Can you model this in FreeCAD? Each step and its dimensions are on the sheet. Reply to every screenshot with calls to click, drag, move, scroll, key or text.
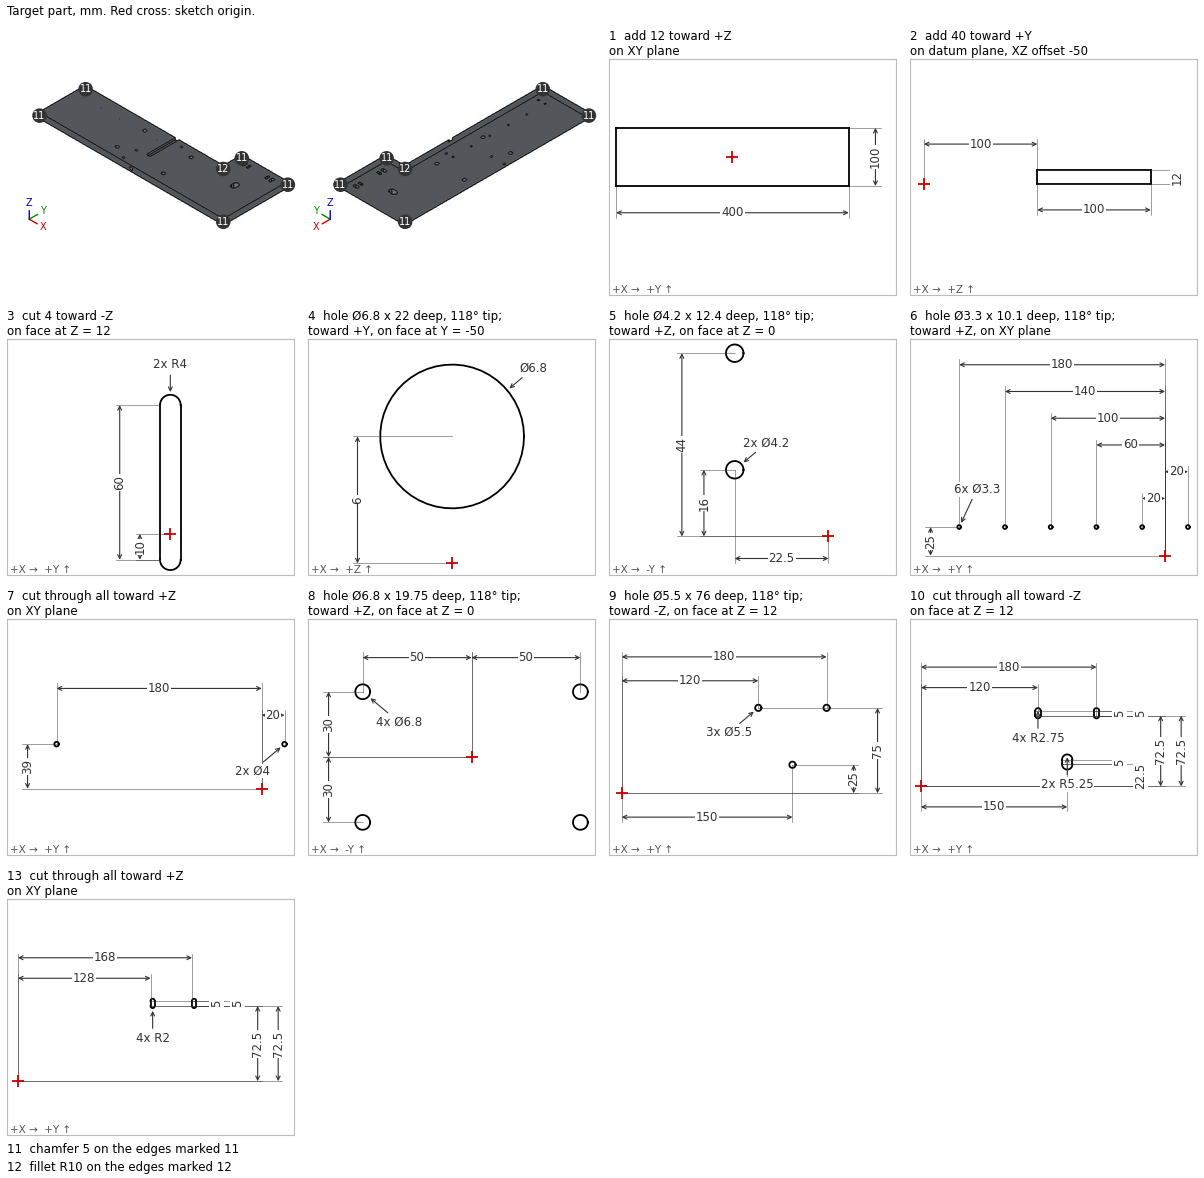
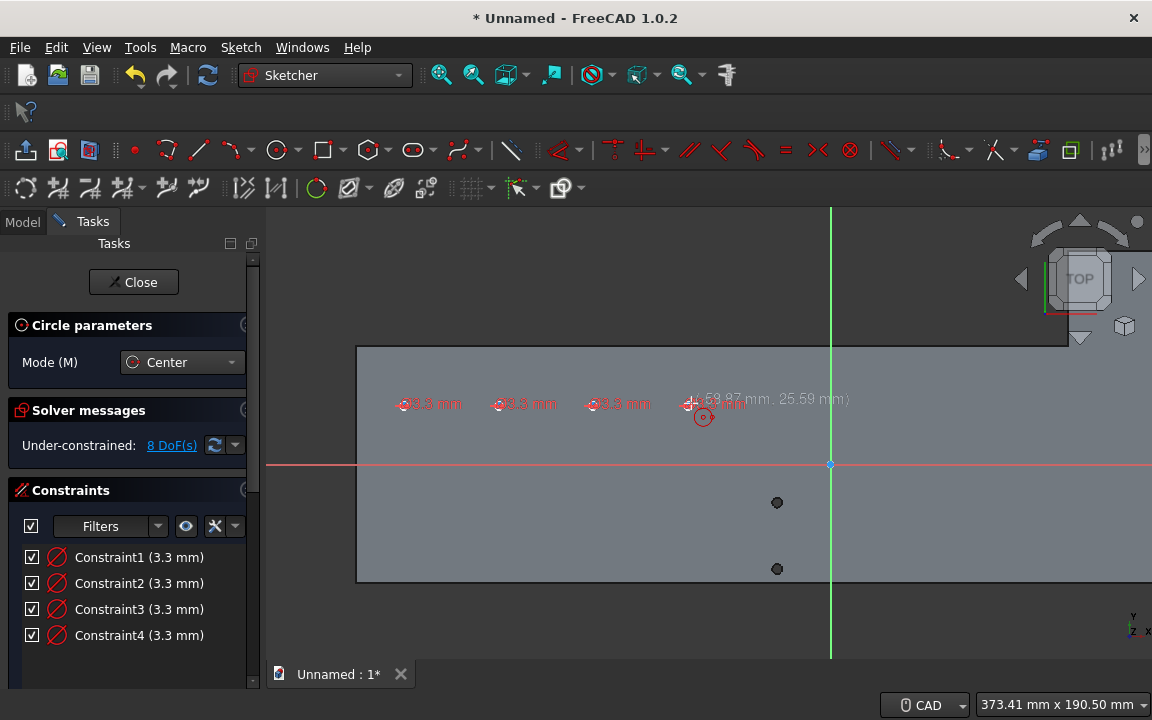
scroll(783, 405, up, 9)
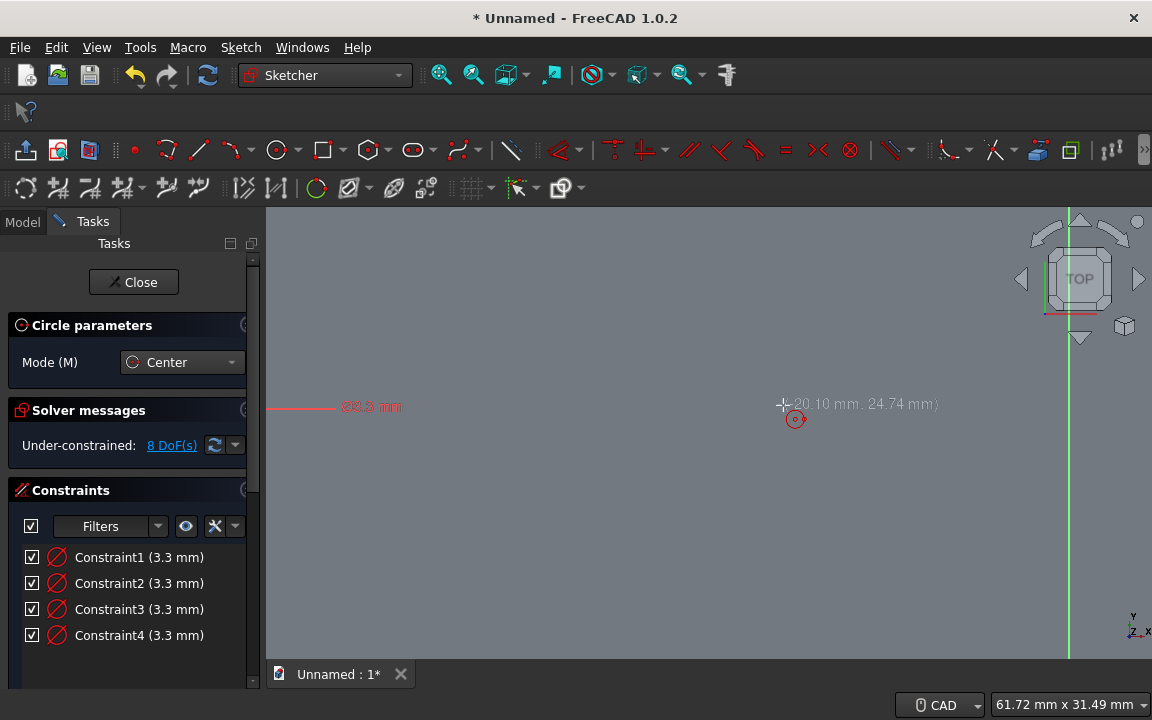
scroll(783, 405, down, 9)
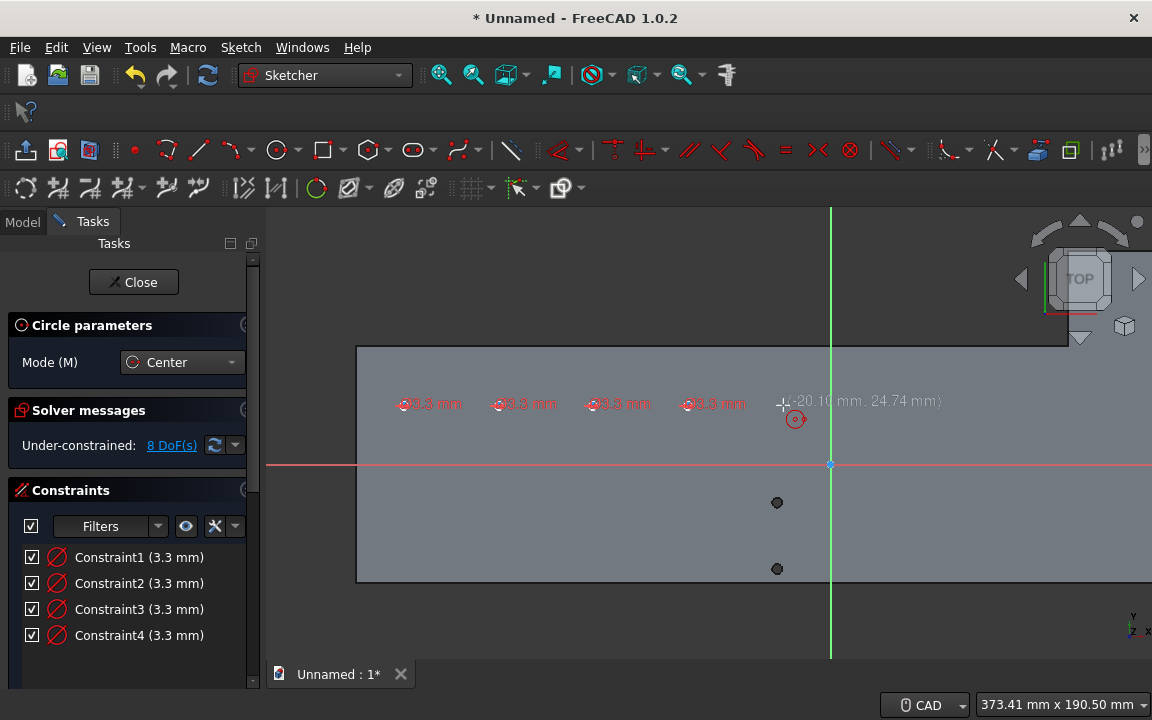
click(783, 405)
move(786, 403)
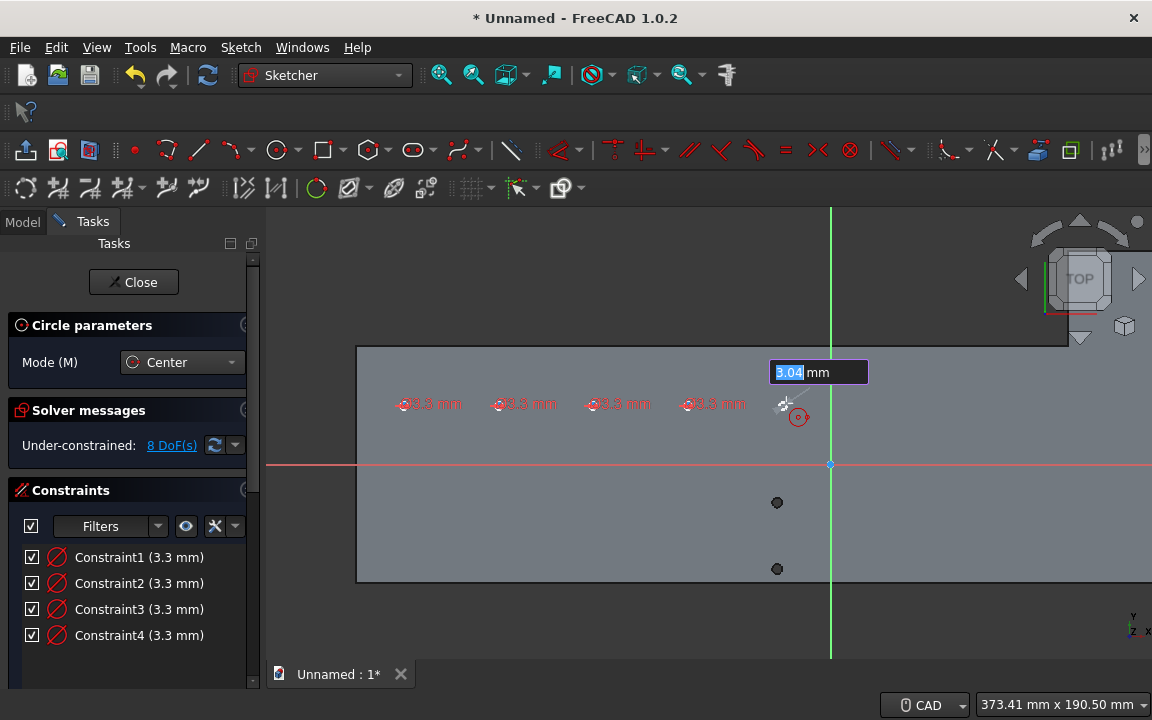
text(3.3)
key(Return)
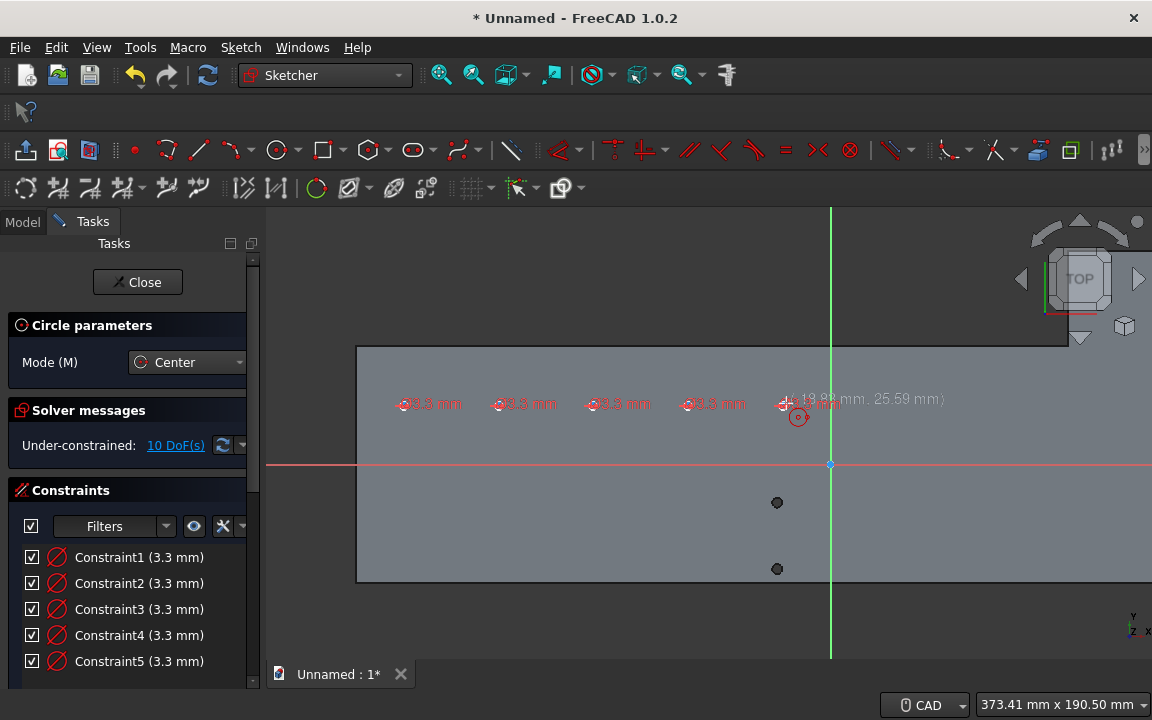
scroll(878, 405, up, 9)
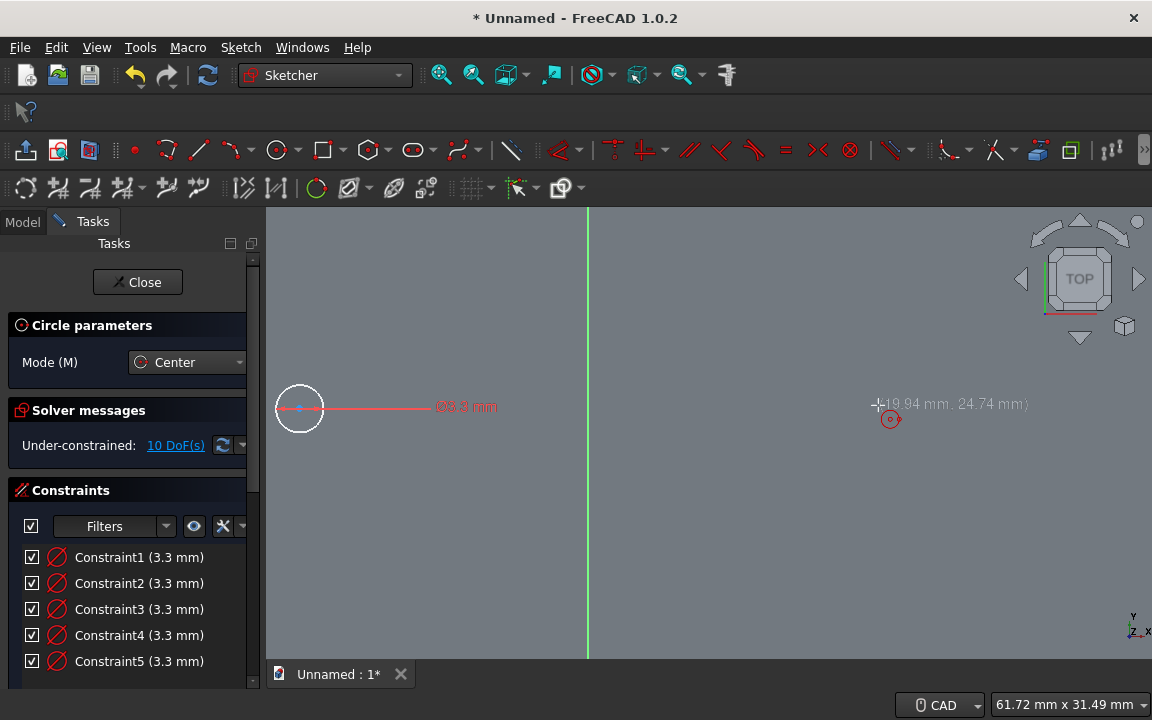
scroll(878, 405, down, 9)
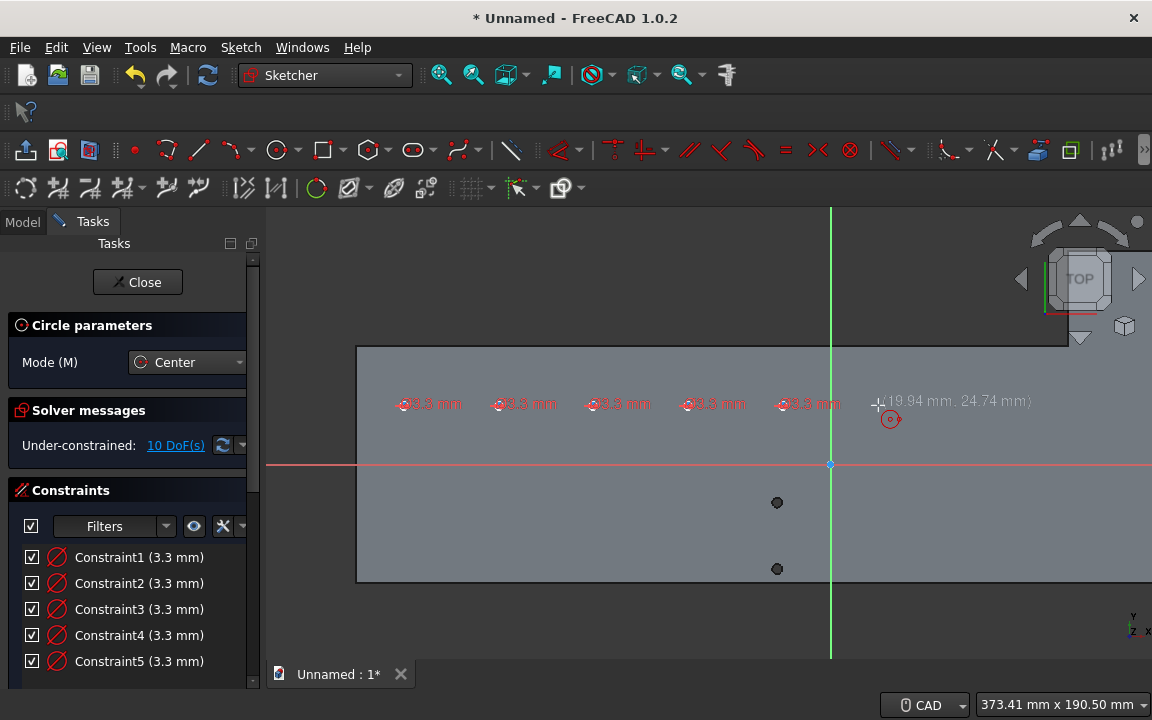
click(878, 405)
move(881, 403)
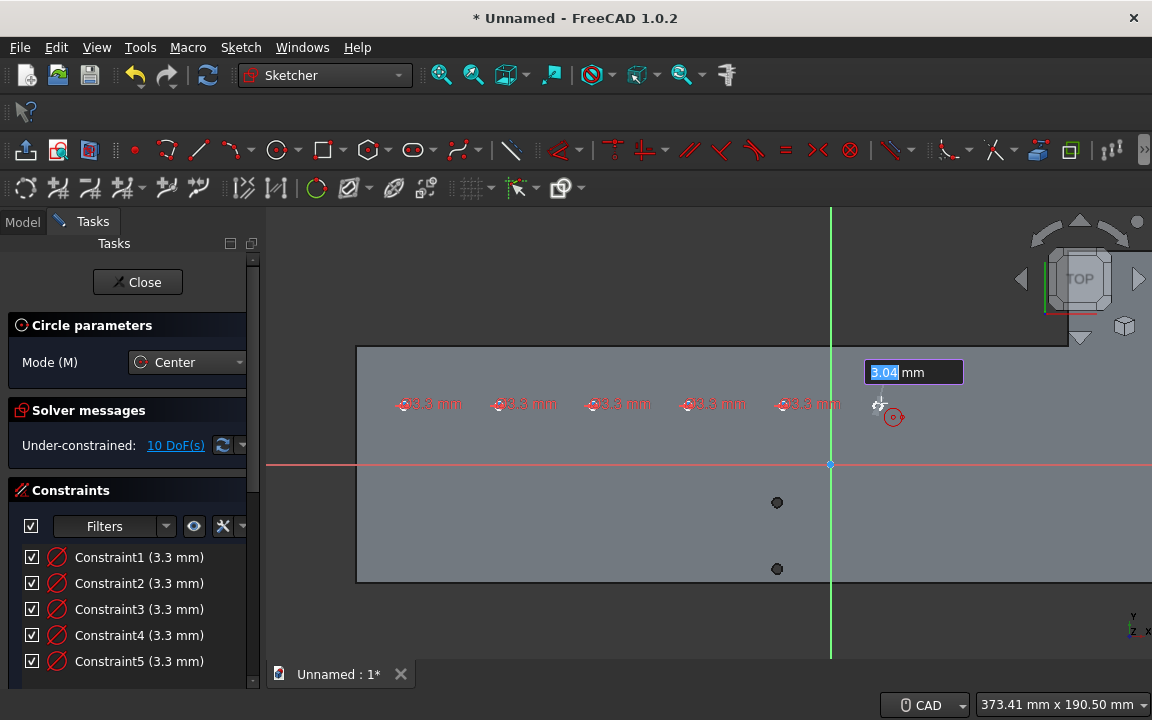
text(3.3)
key(Return)
key(Escape)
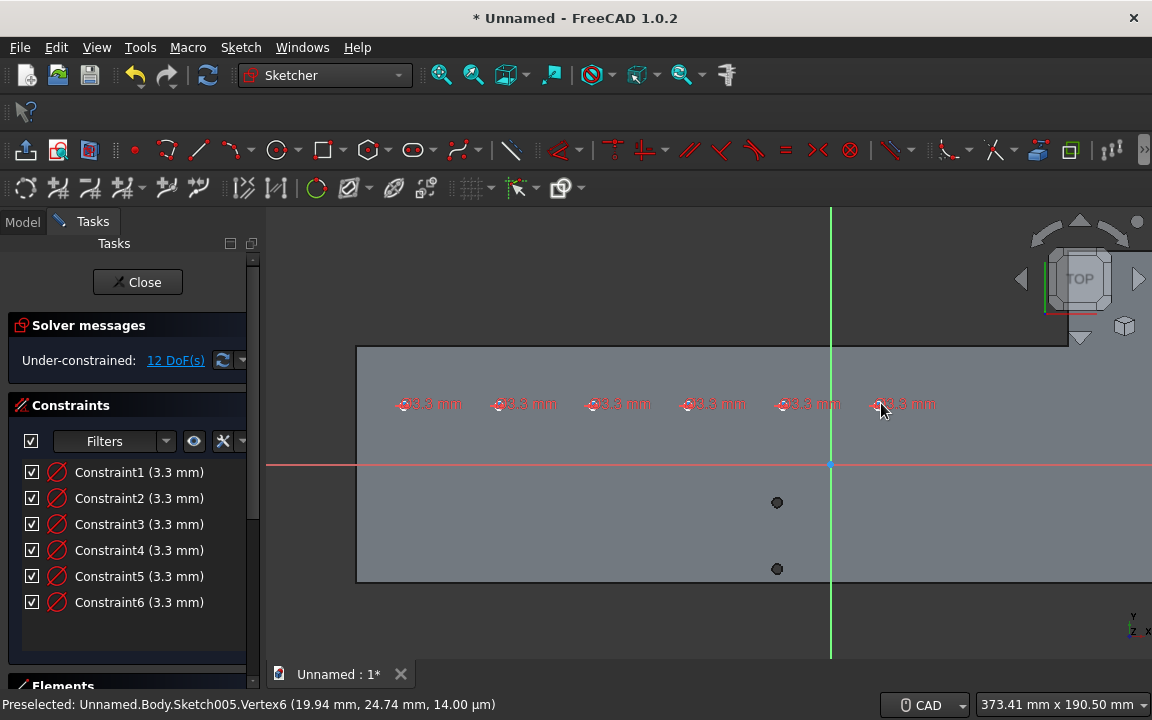
click(404, 406)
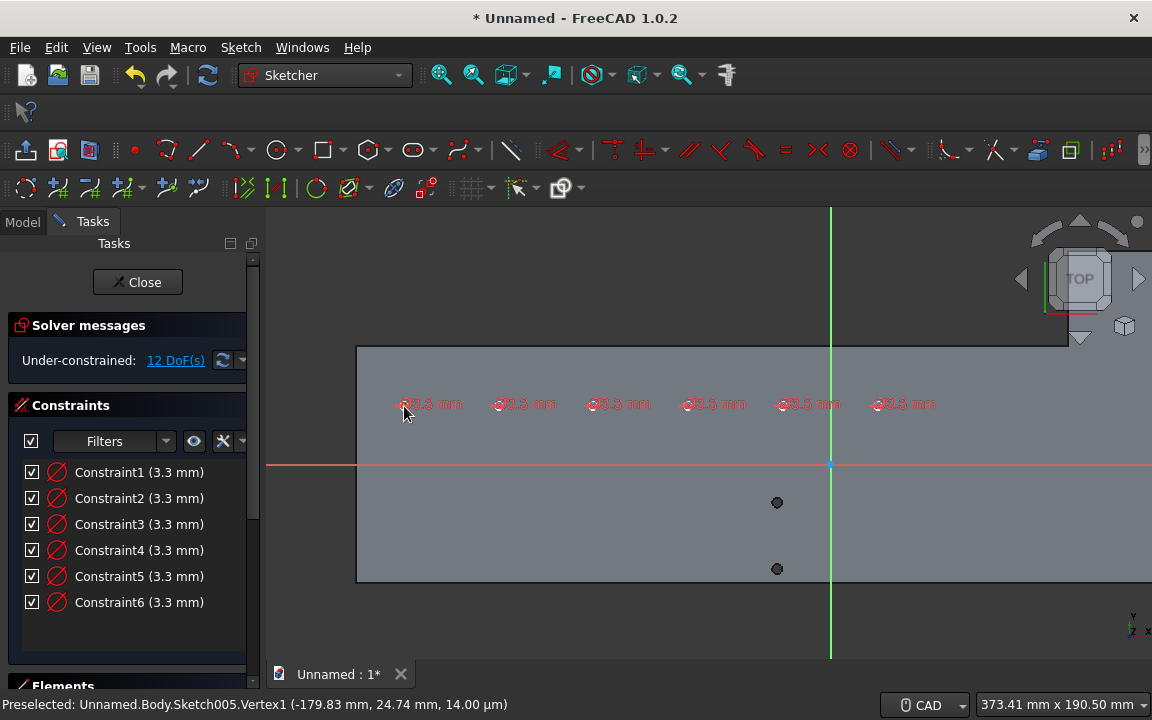
click(499, 406)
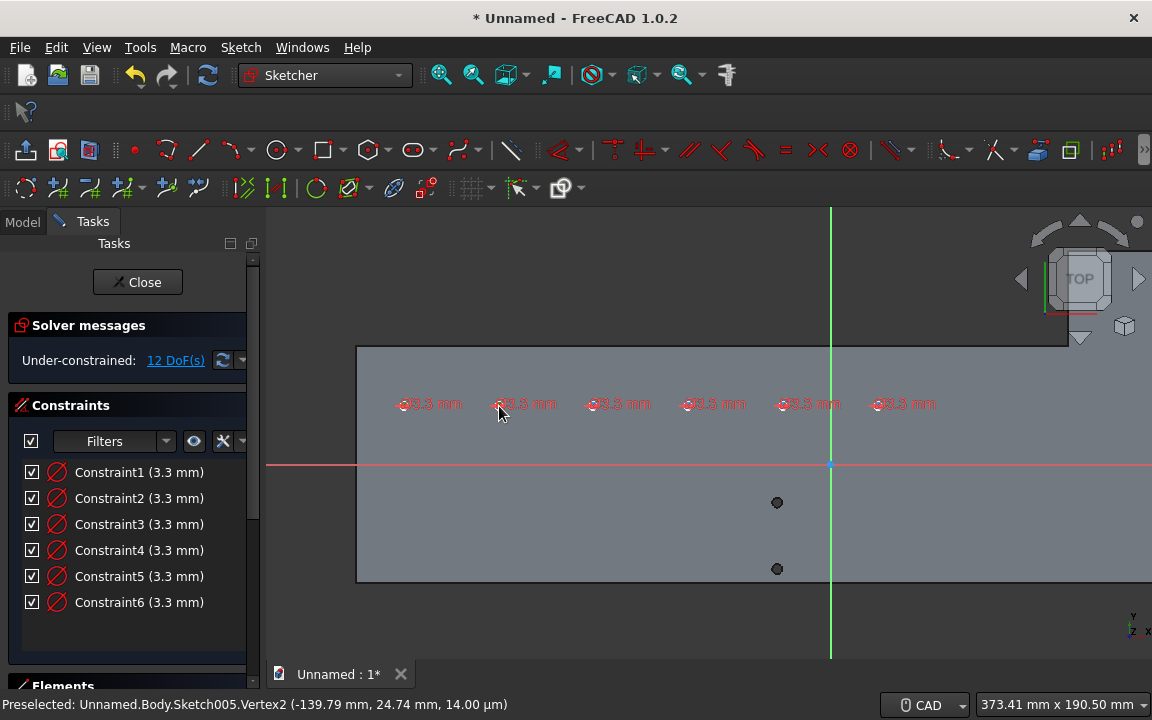
key(h)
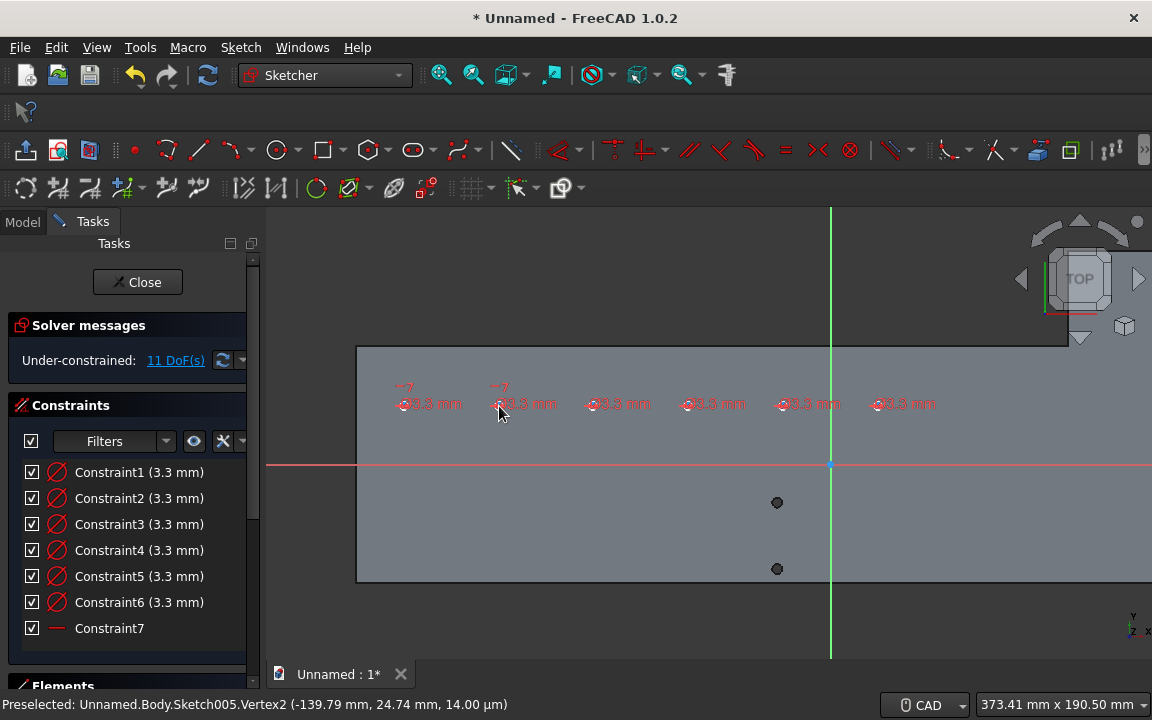
click(499, 406)